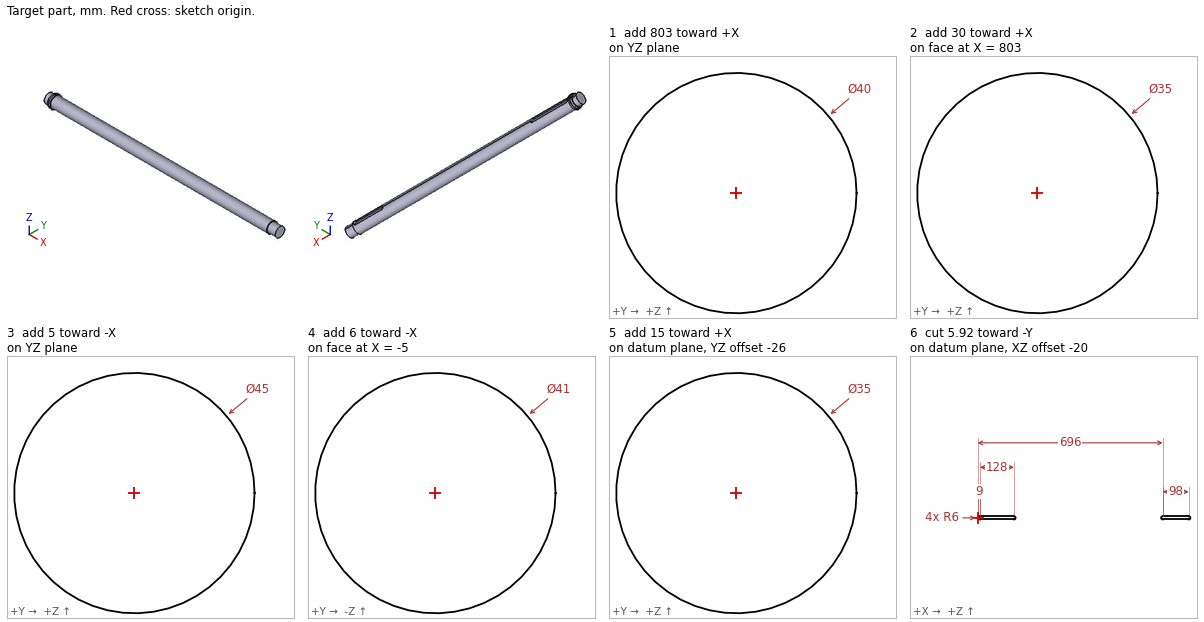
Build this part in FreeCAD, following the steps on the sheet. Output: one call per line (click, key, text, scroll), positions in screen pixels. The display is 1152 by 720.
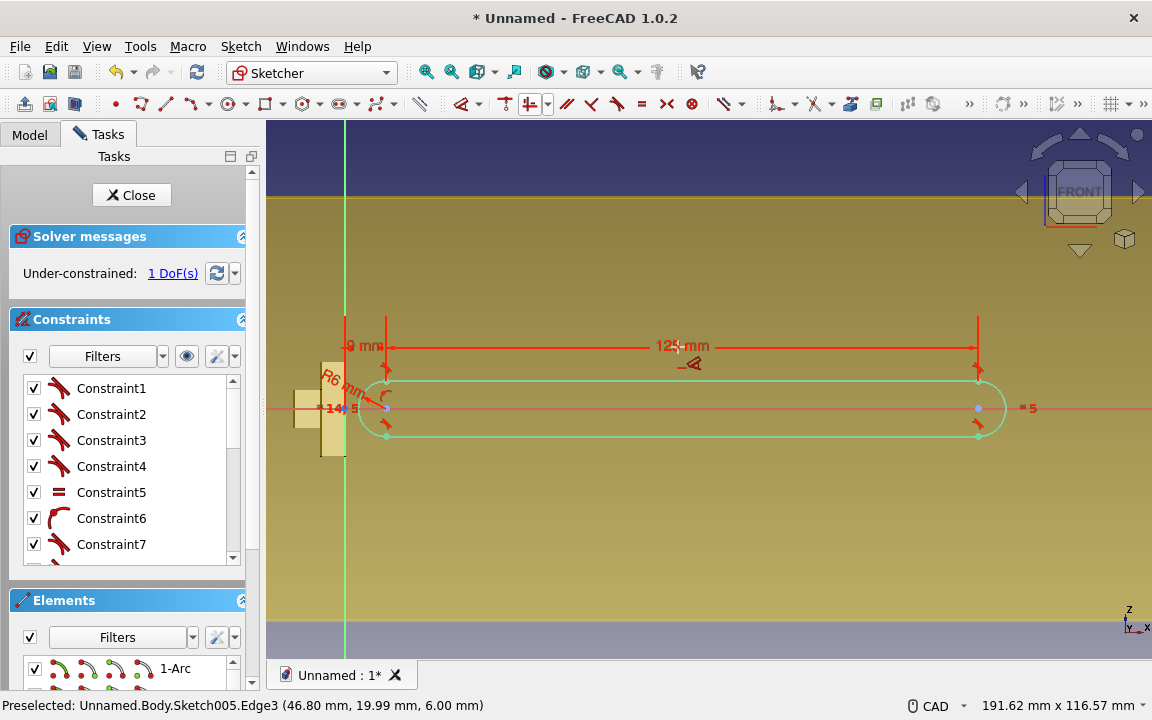
scroll(397, 386, down, 10)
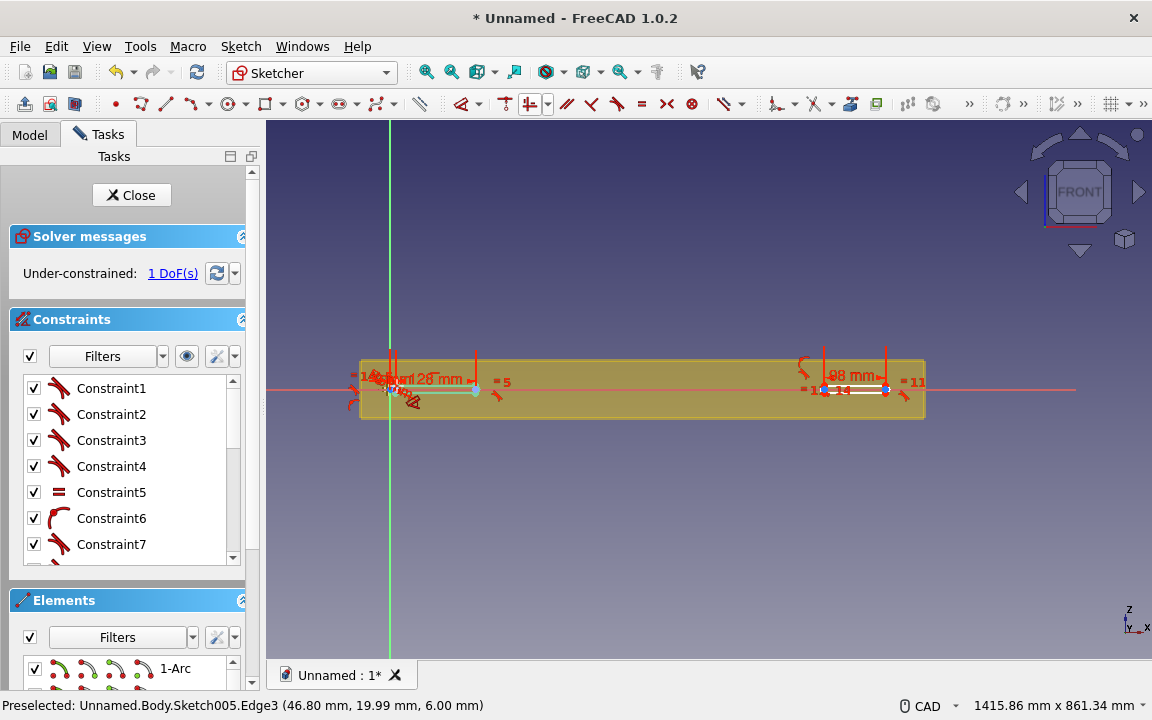
scroll(824, 386, up, 6)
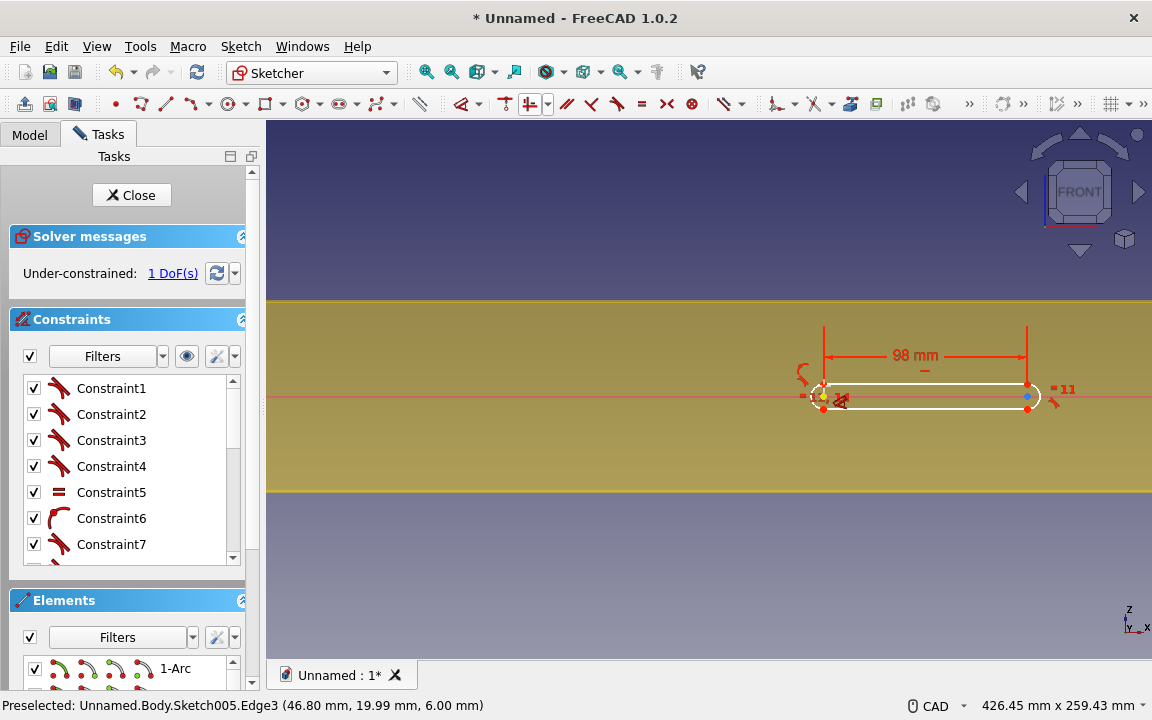
click(824, 384)
click(559, 350)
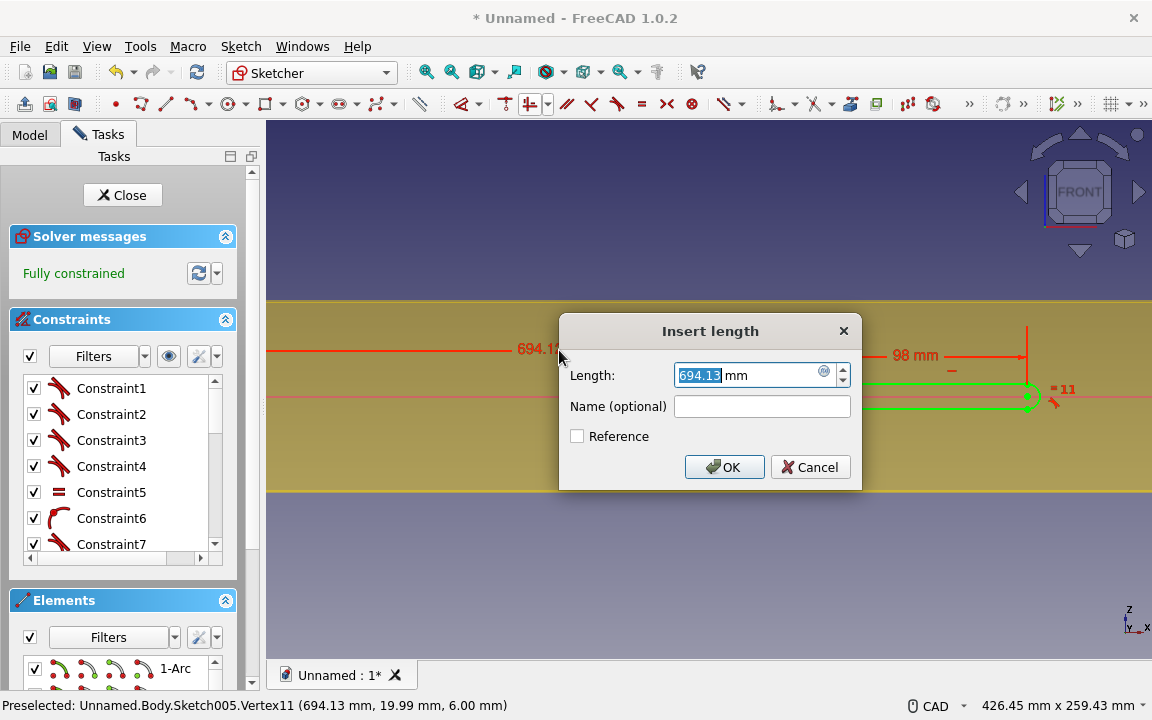
text(696)
key(Return)
key(Escape)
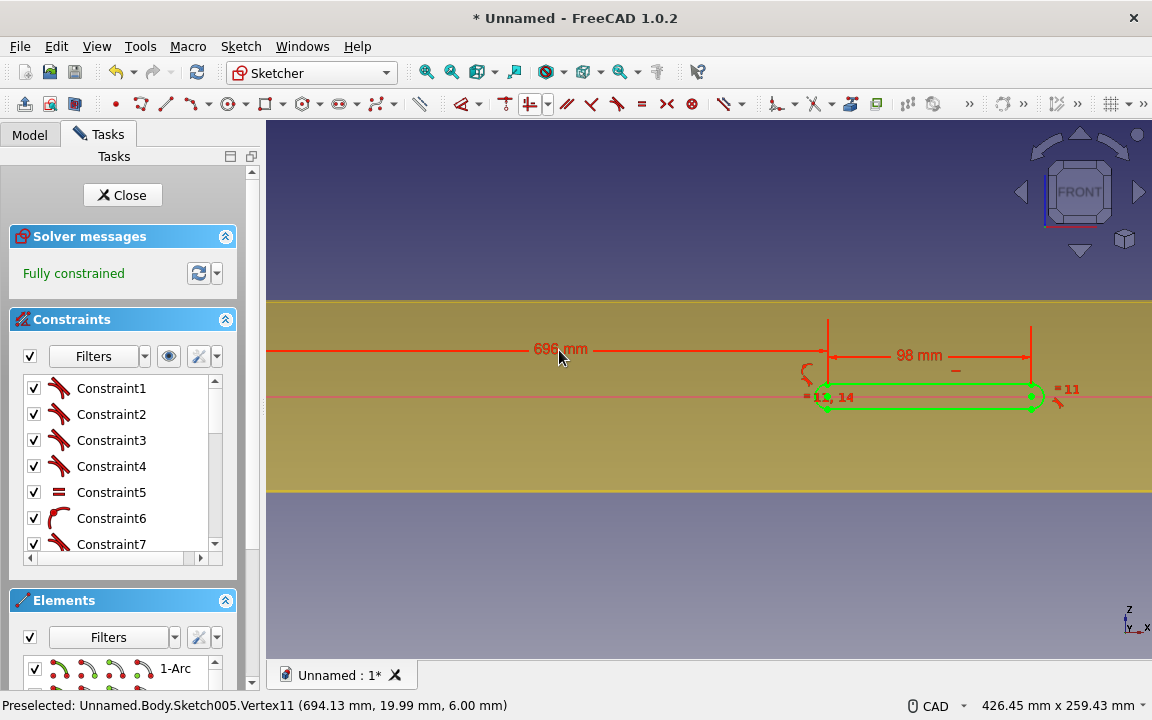
click(123, 195)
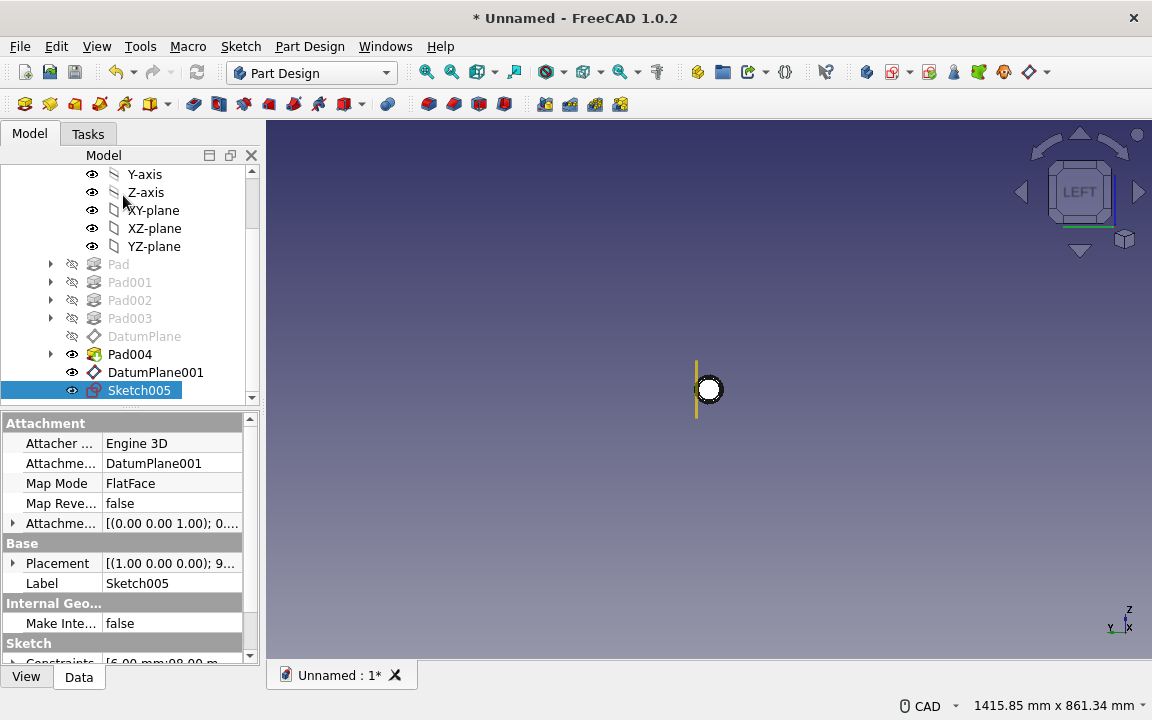
click(194, 104)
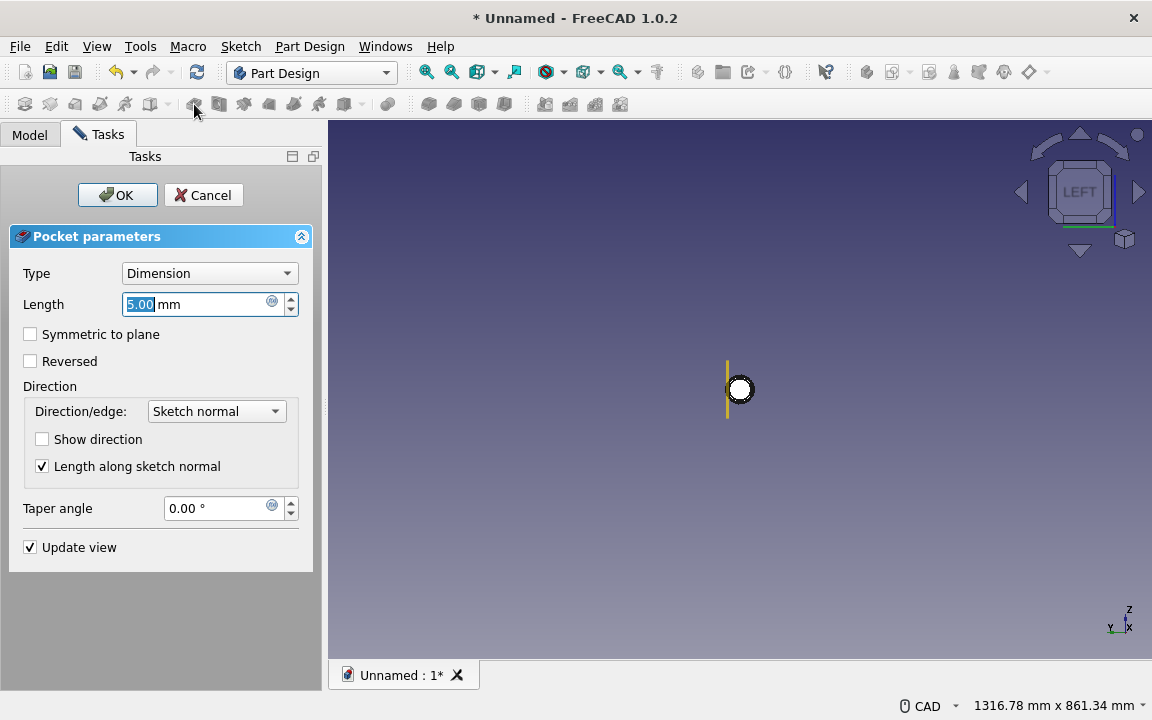
text(5.92)
key(Tab)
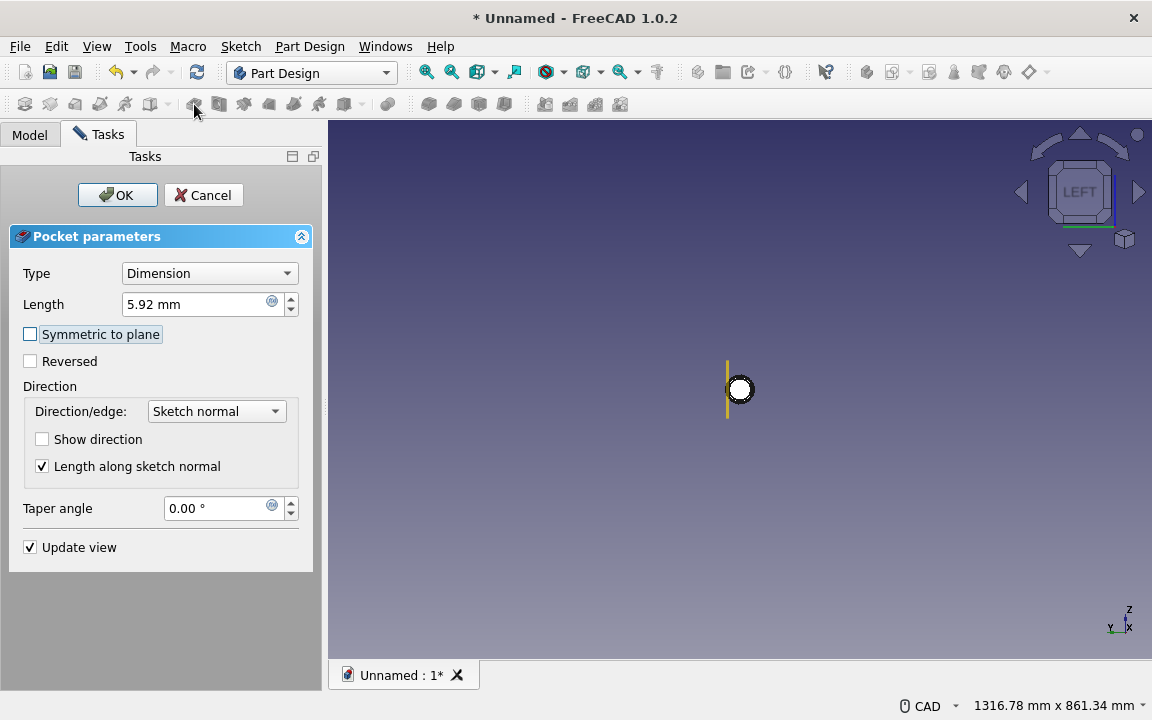
click(31, 361)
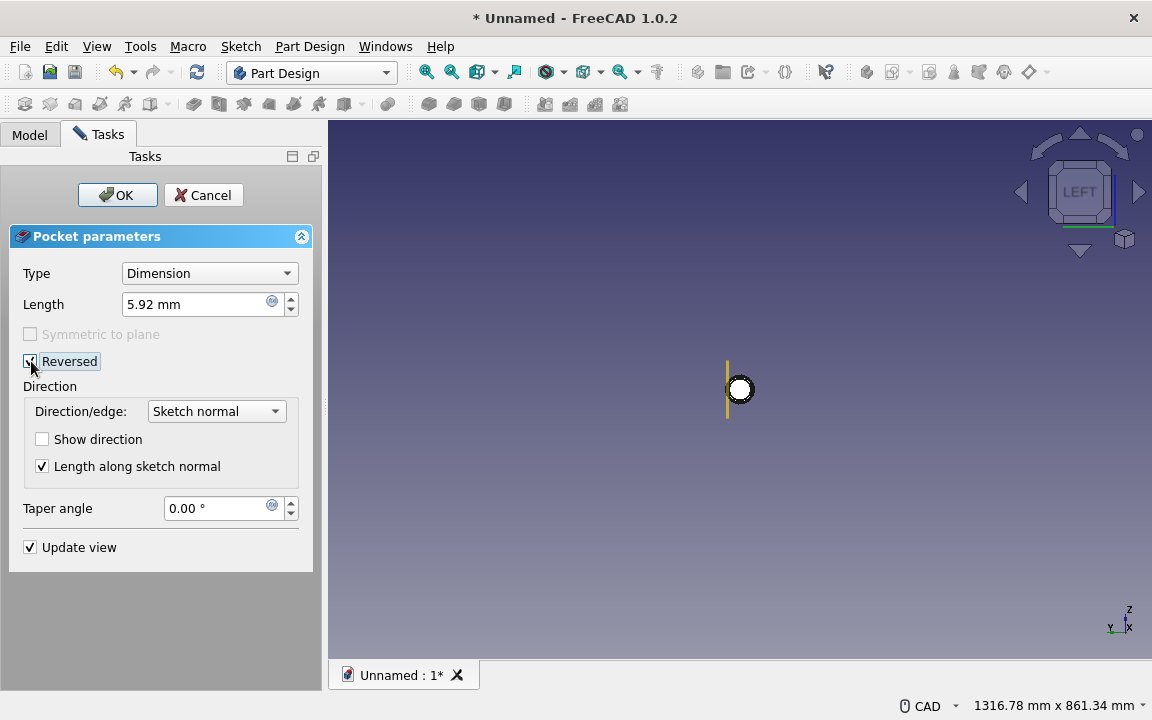
click(118, 195)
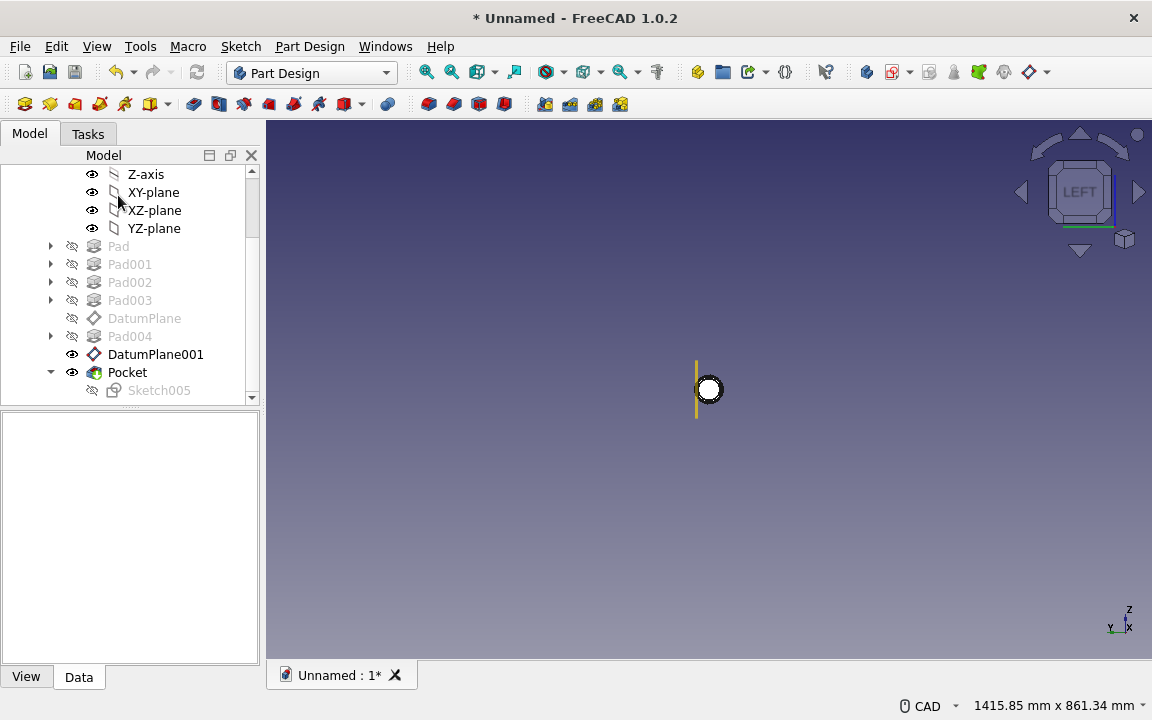
click(117, 354)
key(space)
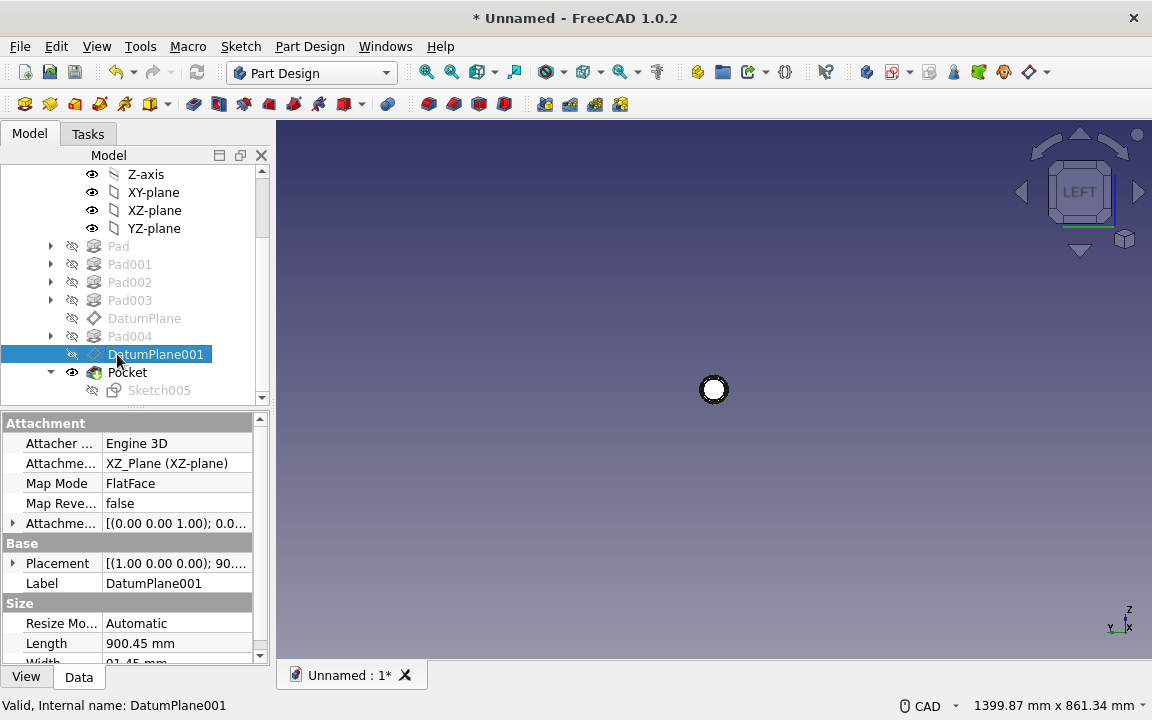
key(0)